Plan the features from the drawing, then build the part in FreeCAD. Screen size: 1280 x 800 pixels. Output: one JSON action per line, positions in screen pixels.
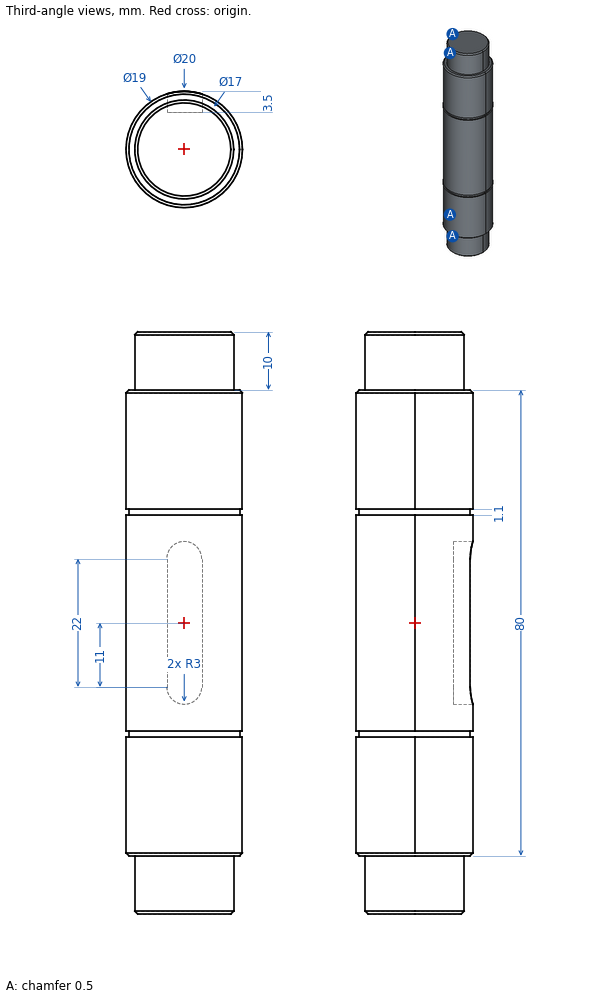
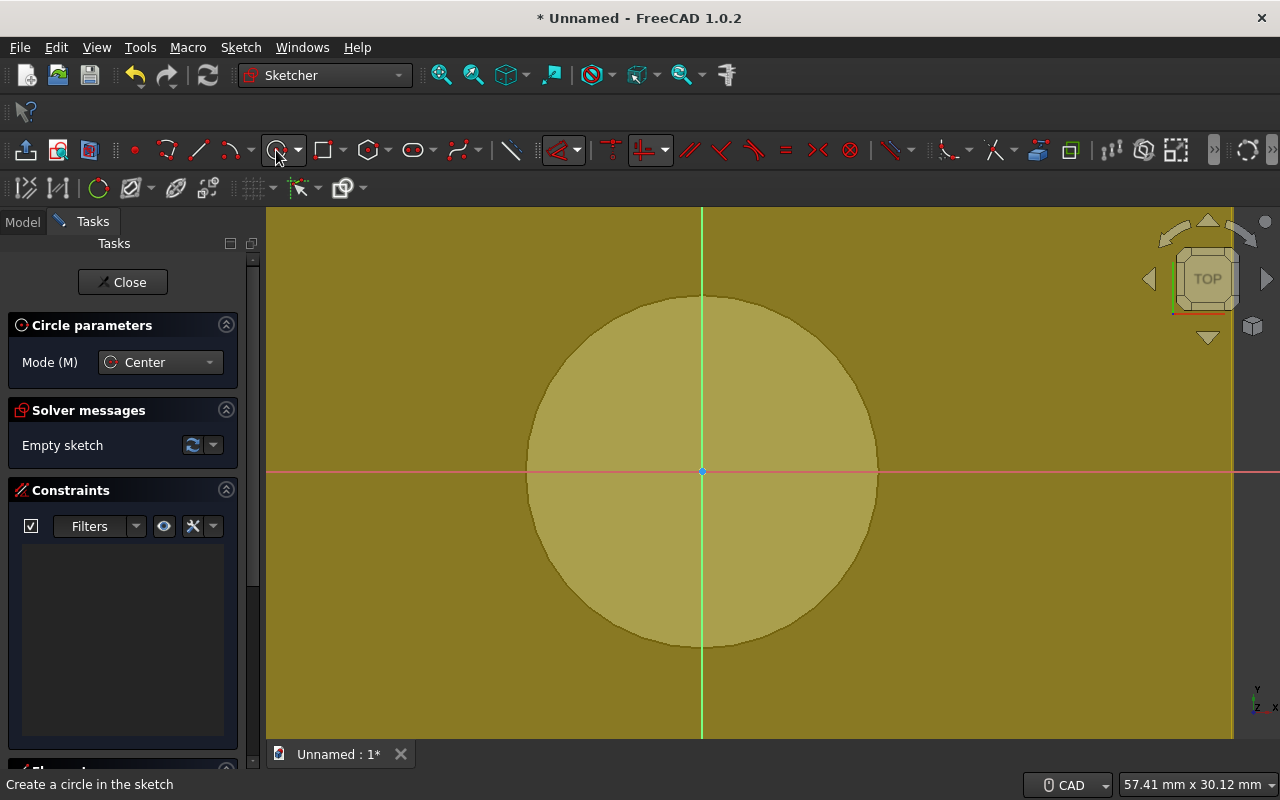
{"action": "left_click", "coordinate": [702, 472]}
{"action": "left_click", "coordinate": [827, 347]}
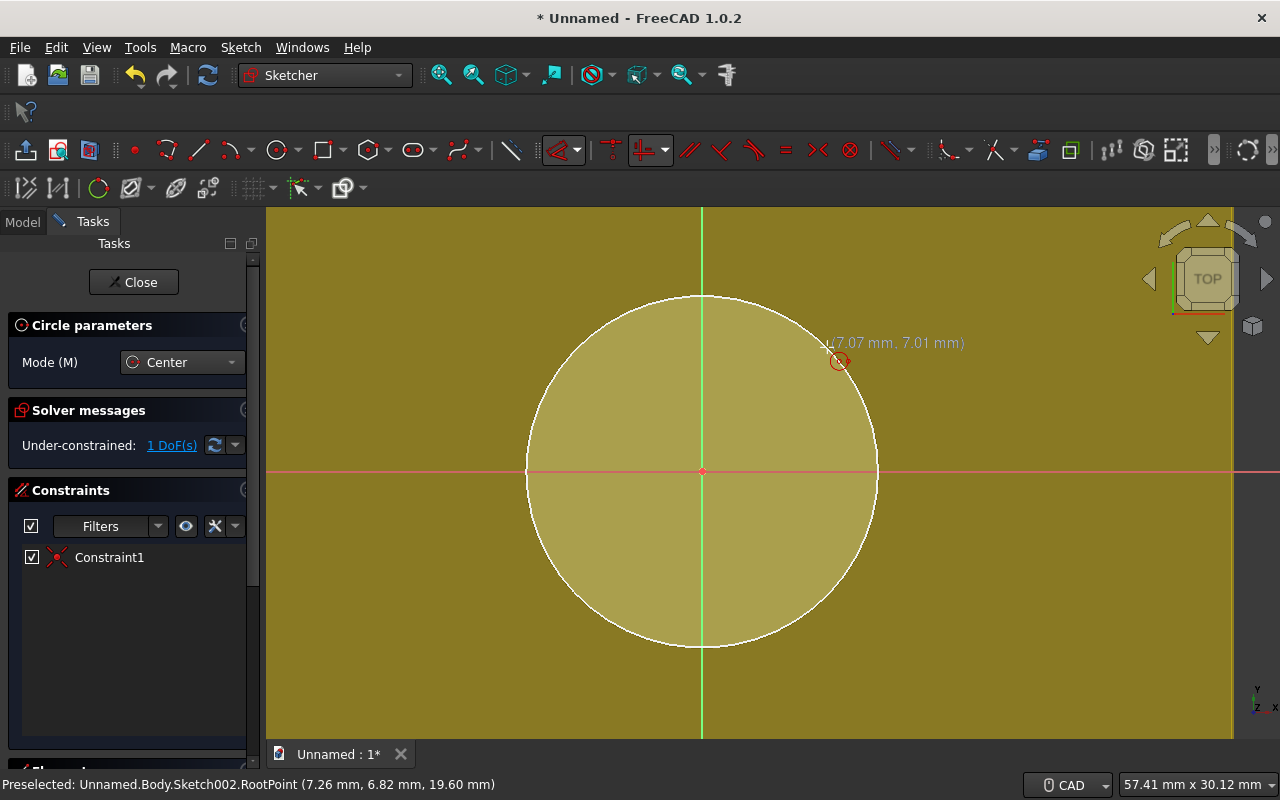
{"action": "left_click", "coordinate": [702, 472]}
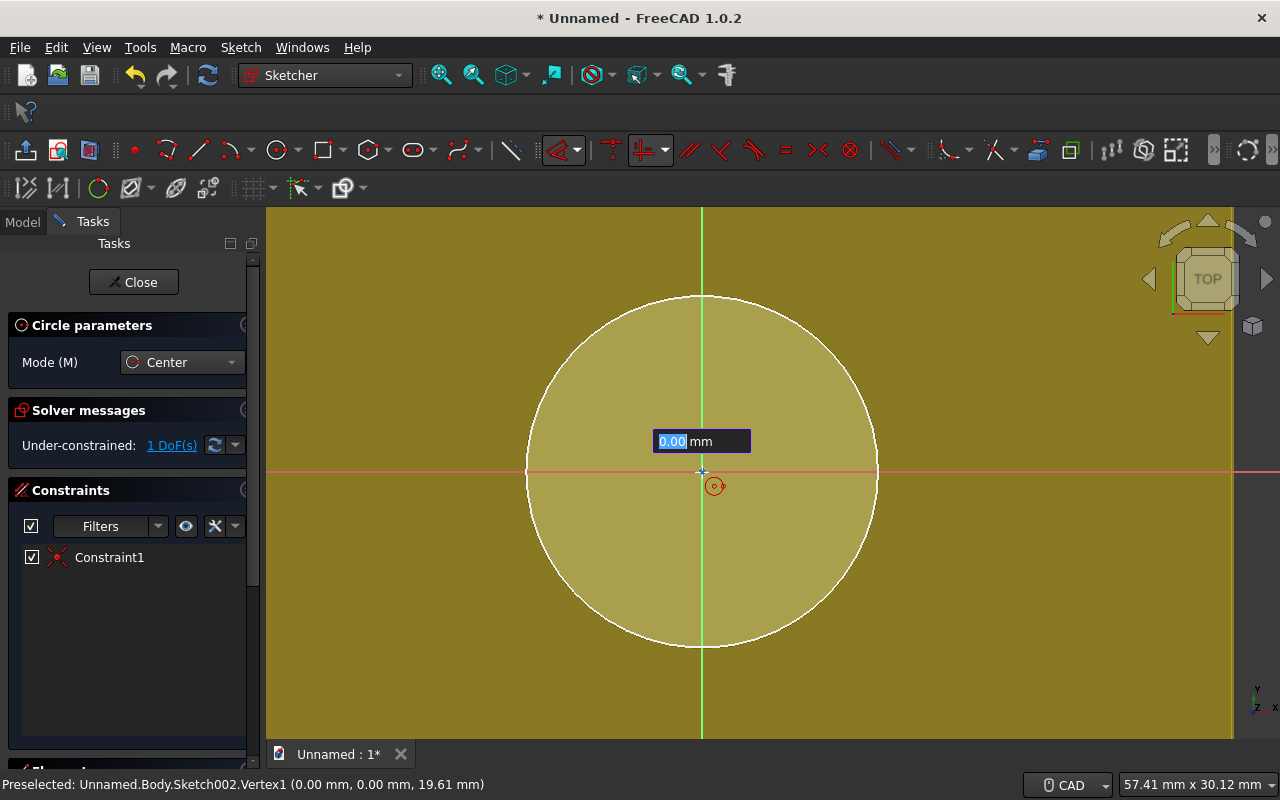
{"action": "scroll", "coordinate": [821, 353], "scroll_direction": "up", "scroll_amount": 3}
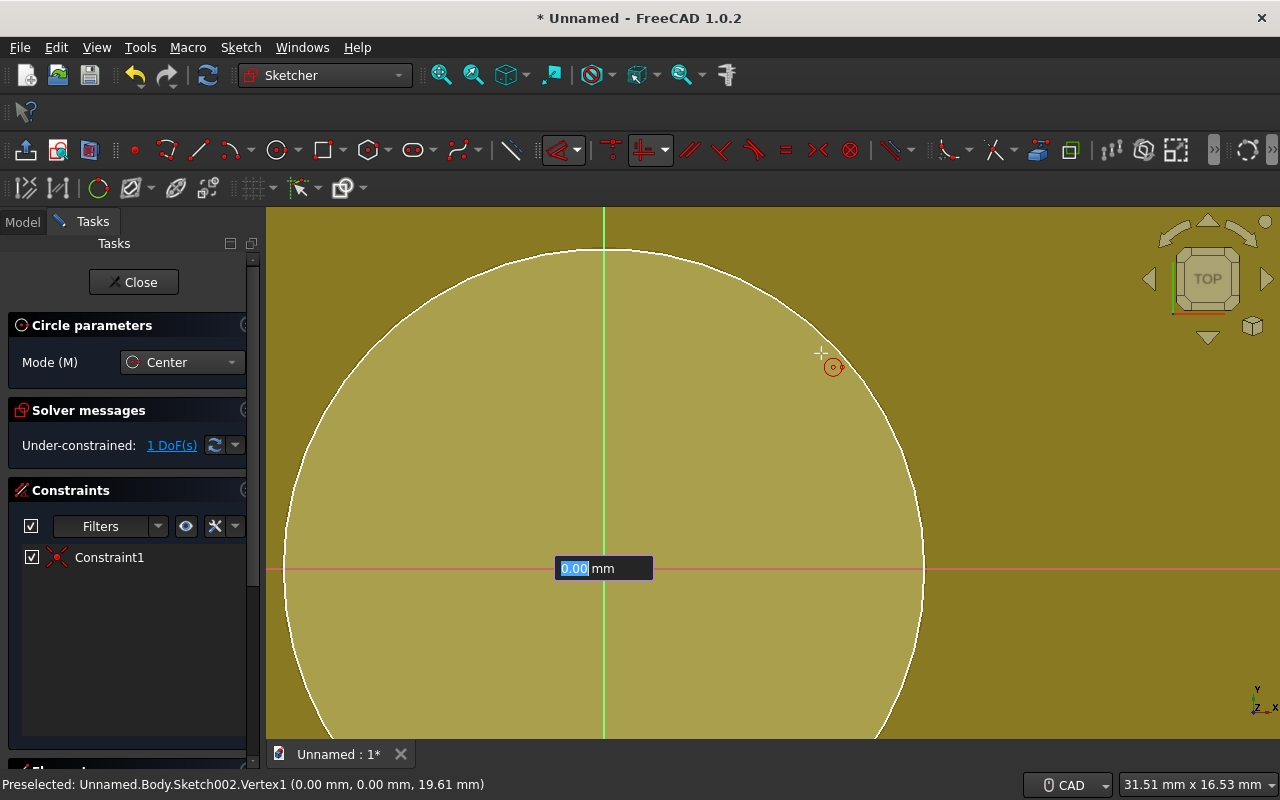
{"action": "left_click", "coordinate": [820, 353]}
{"action": "key", "text": "Escape"}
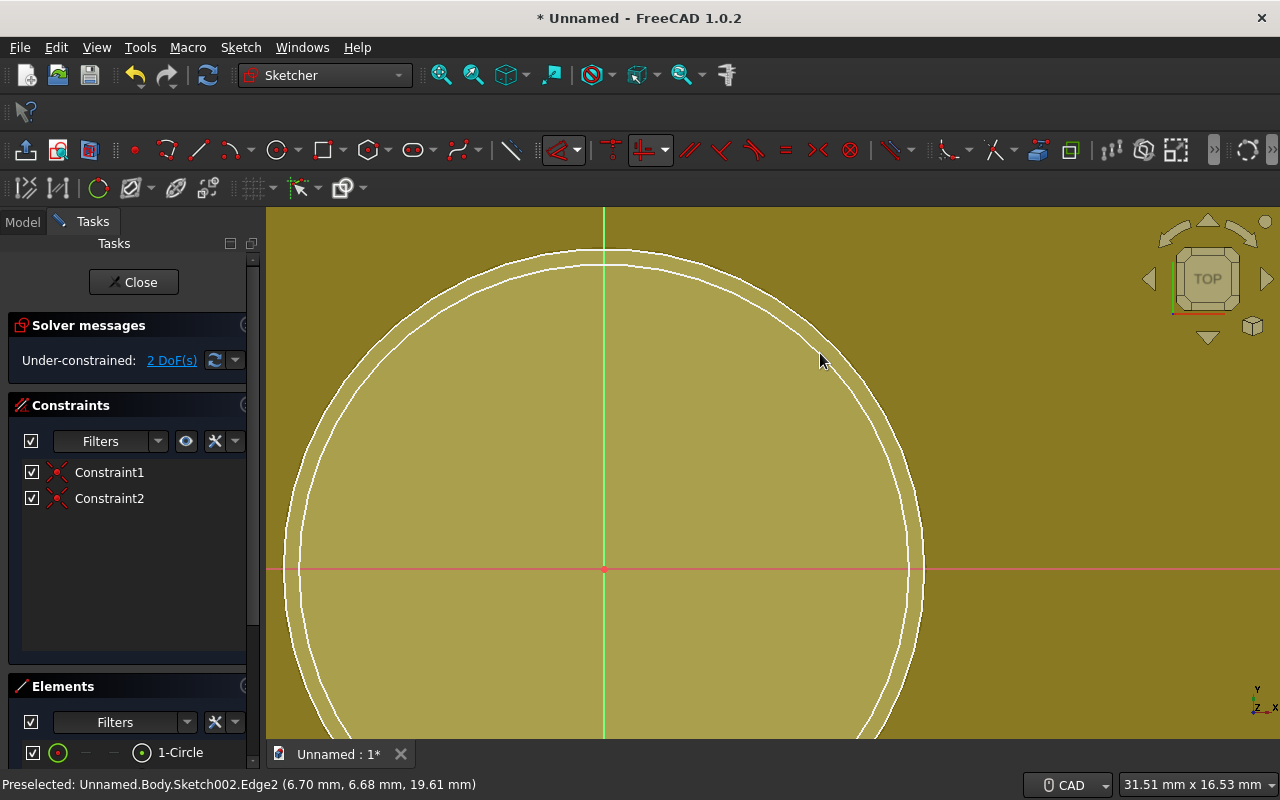
{"action": "key", "text": "d"}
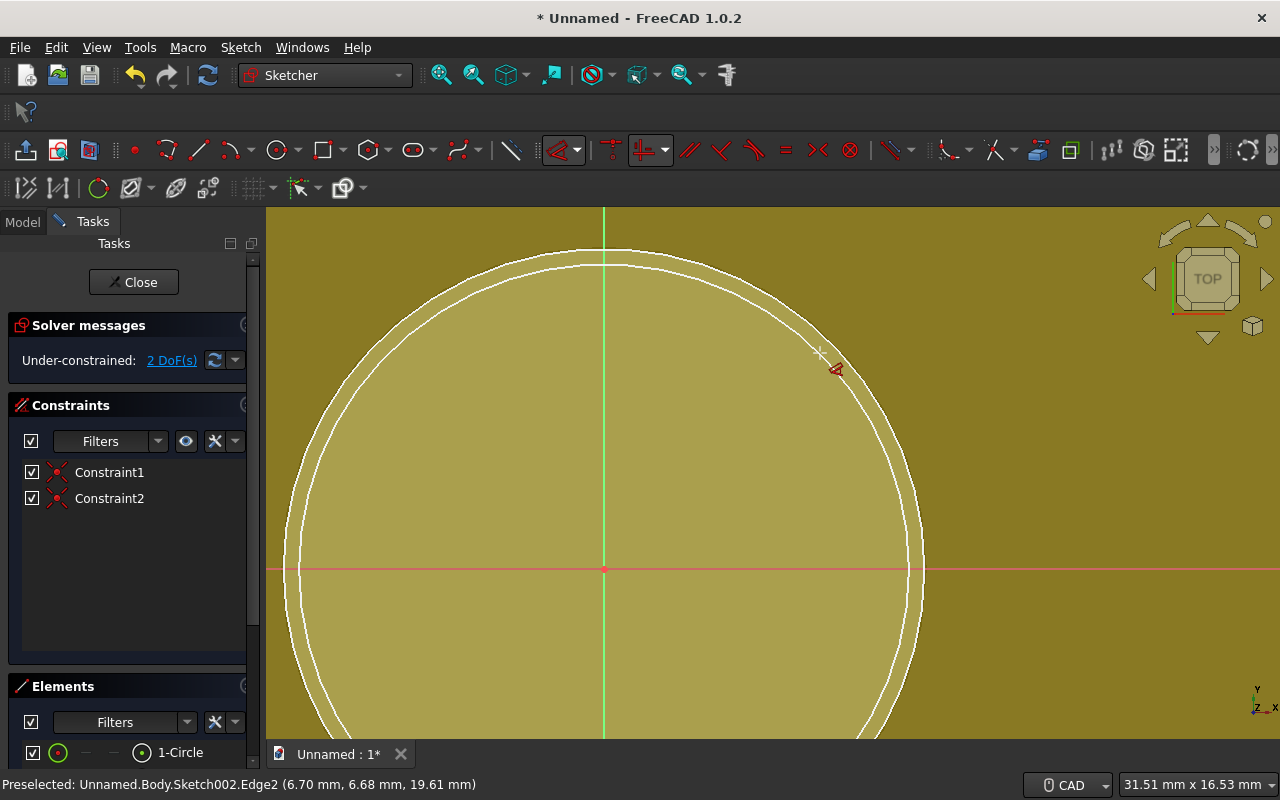
{"action": "left_click", "coordinate": [830, 342]}
{"action": "left_click", "coordinate": [853, 319]}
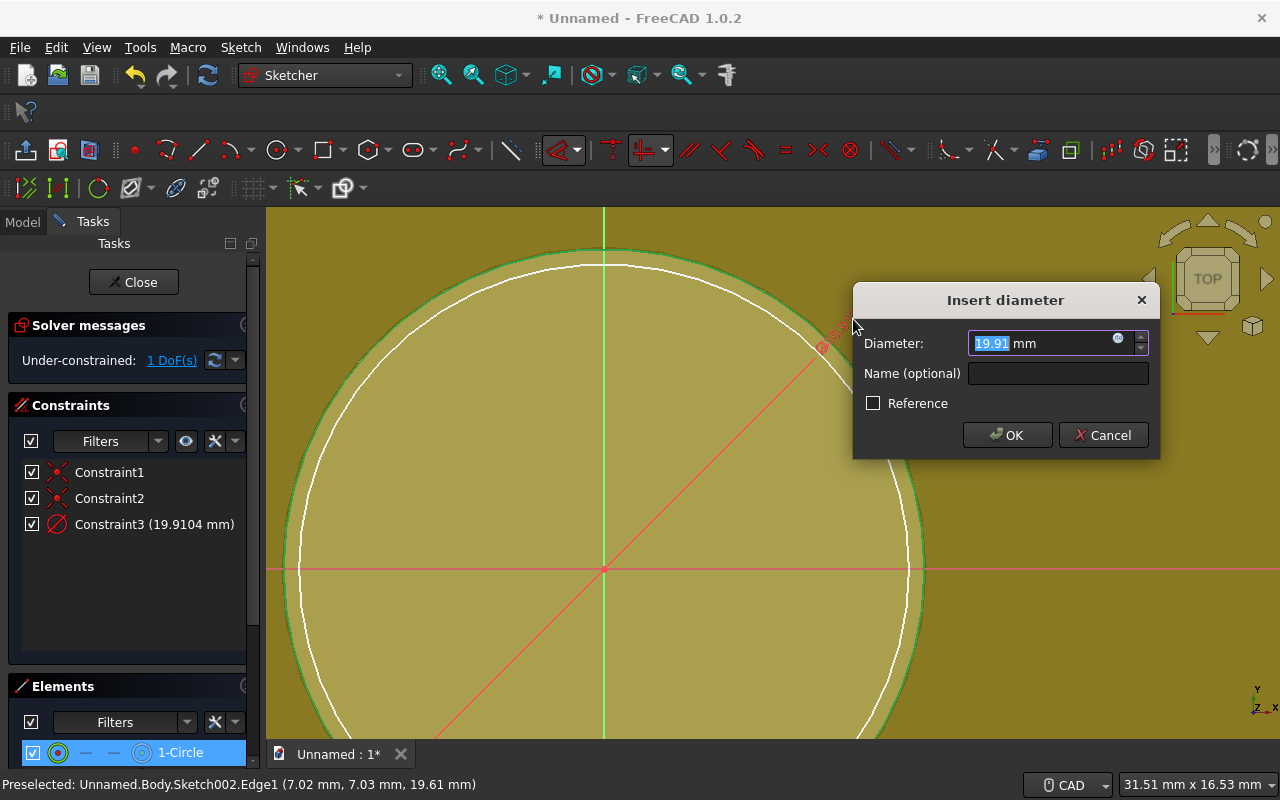
{"action": "type", "text": "20"}
{"action": "key", "text": "Return"}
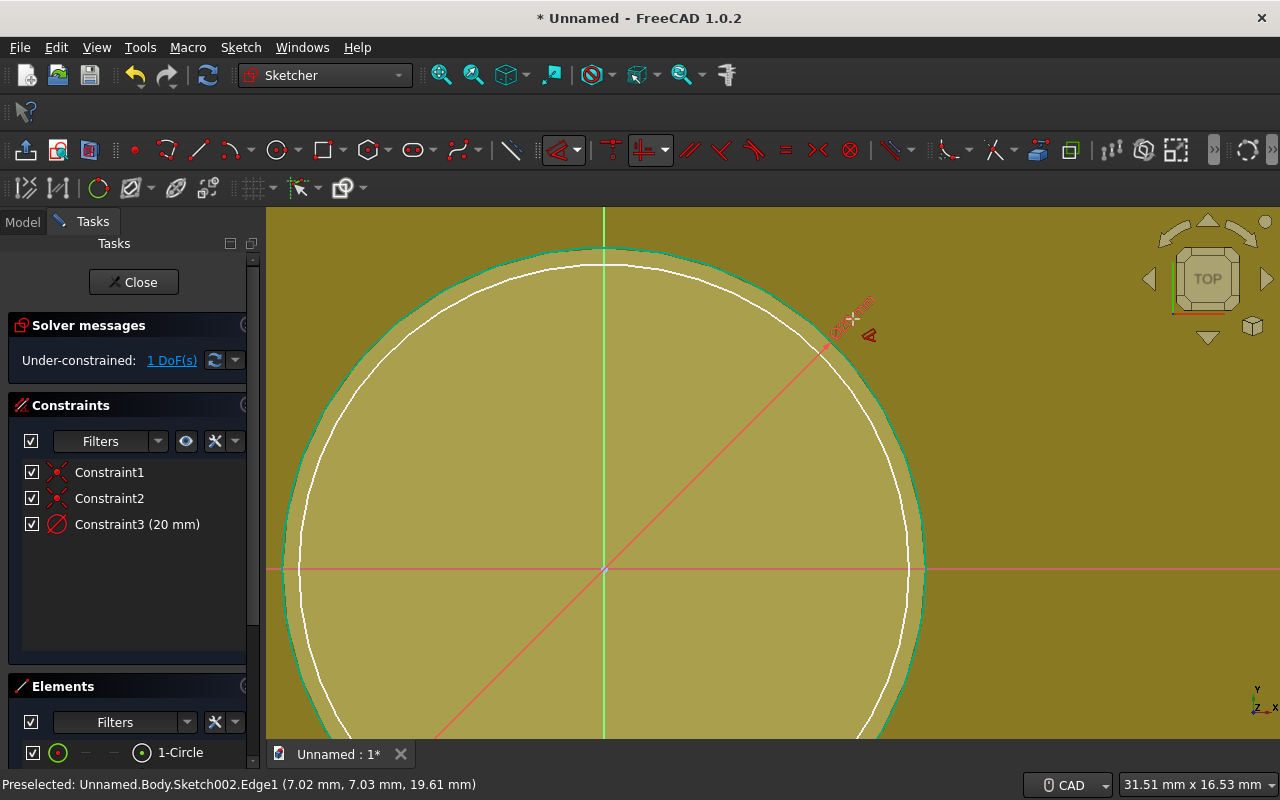
{"action": "left_click", "coordinate": [819, 353]}
{"action": "left_click", "coordinate": [927, 473]}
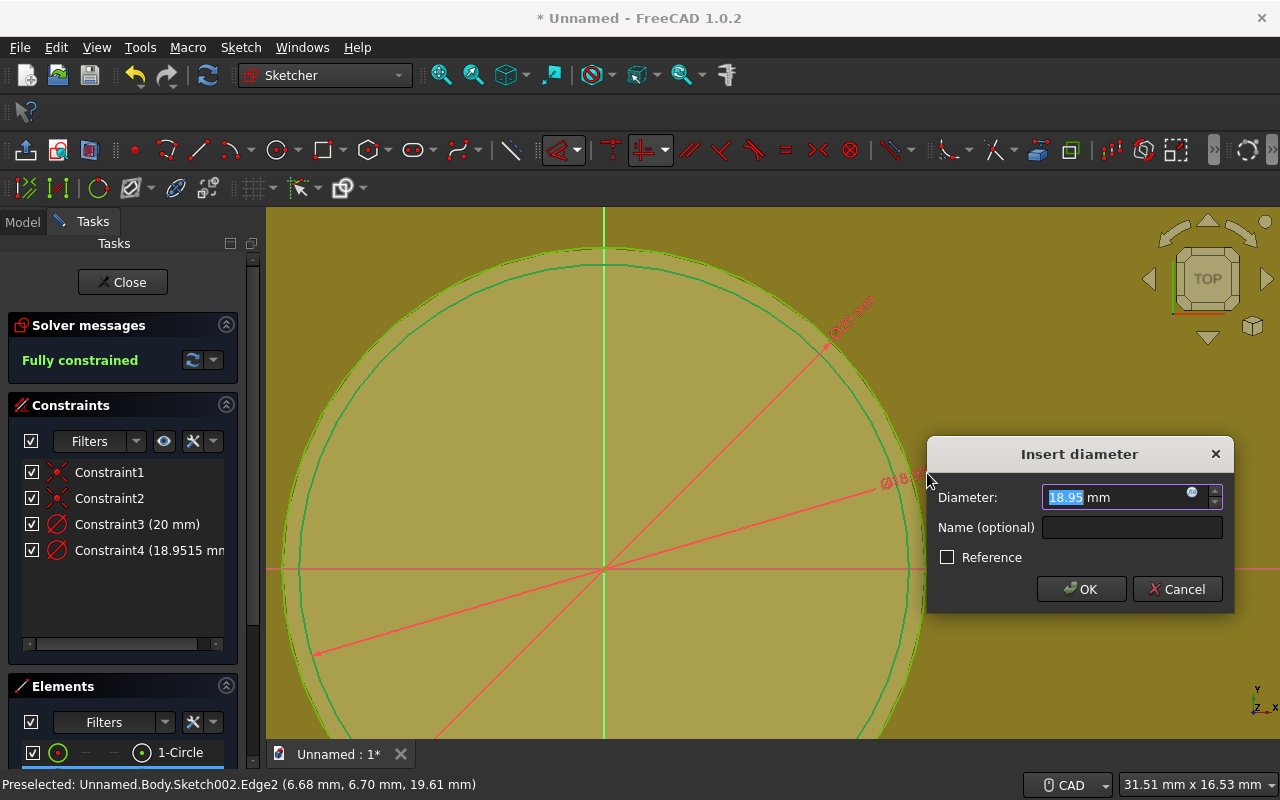
{"action": "type", "text": "19"}
{"action": "key", "text": "Return"}
{"action": "key", "text": "Escape"}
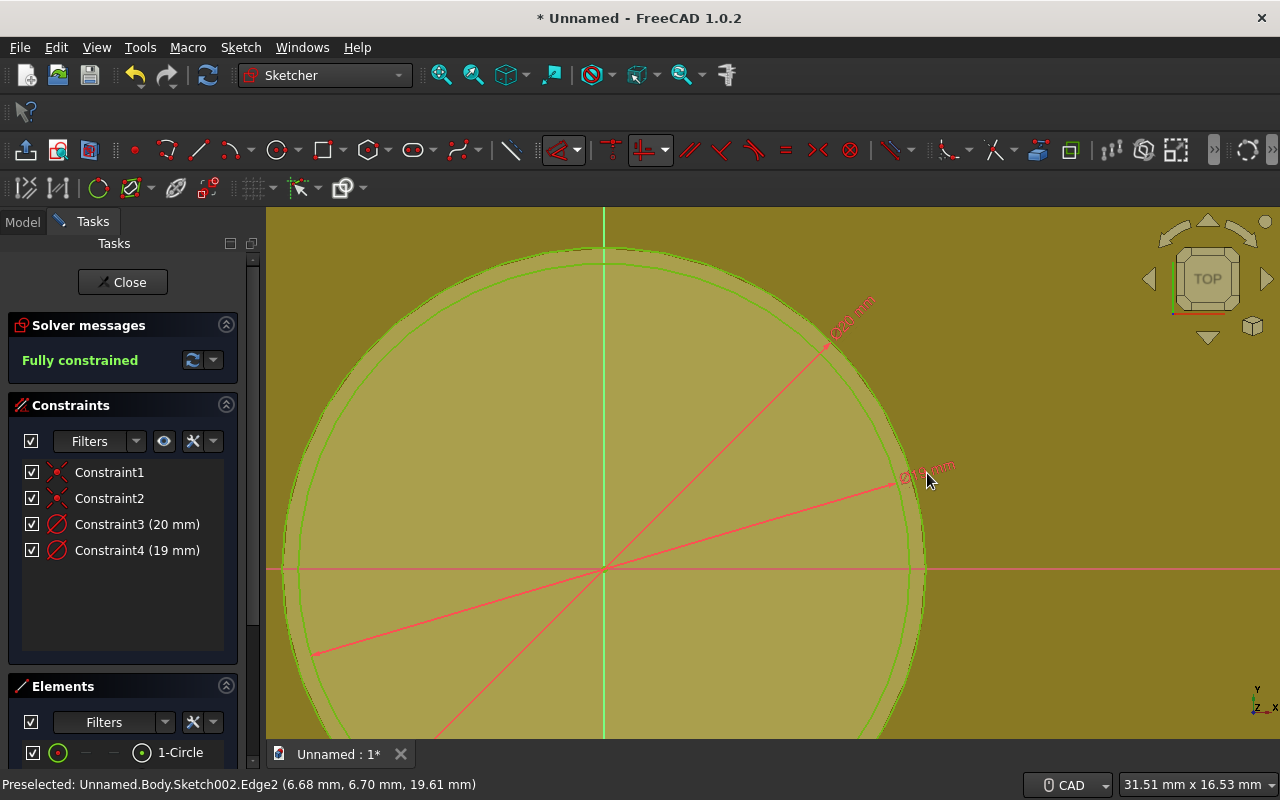
{"action": "left_click", "coordinate": [123, 282]}